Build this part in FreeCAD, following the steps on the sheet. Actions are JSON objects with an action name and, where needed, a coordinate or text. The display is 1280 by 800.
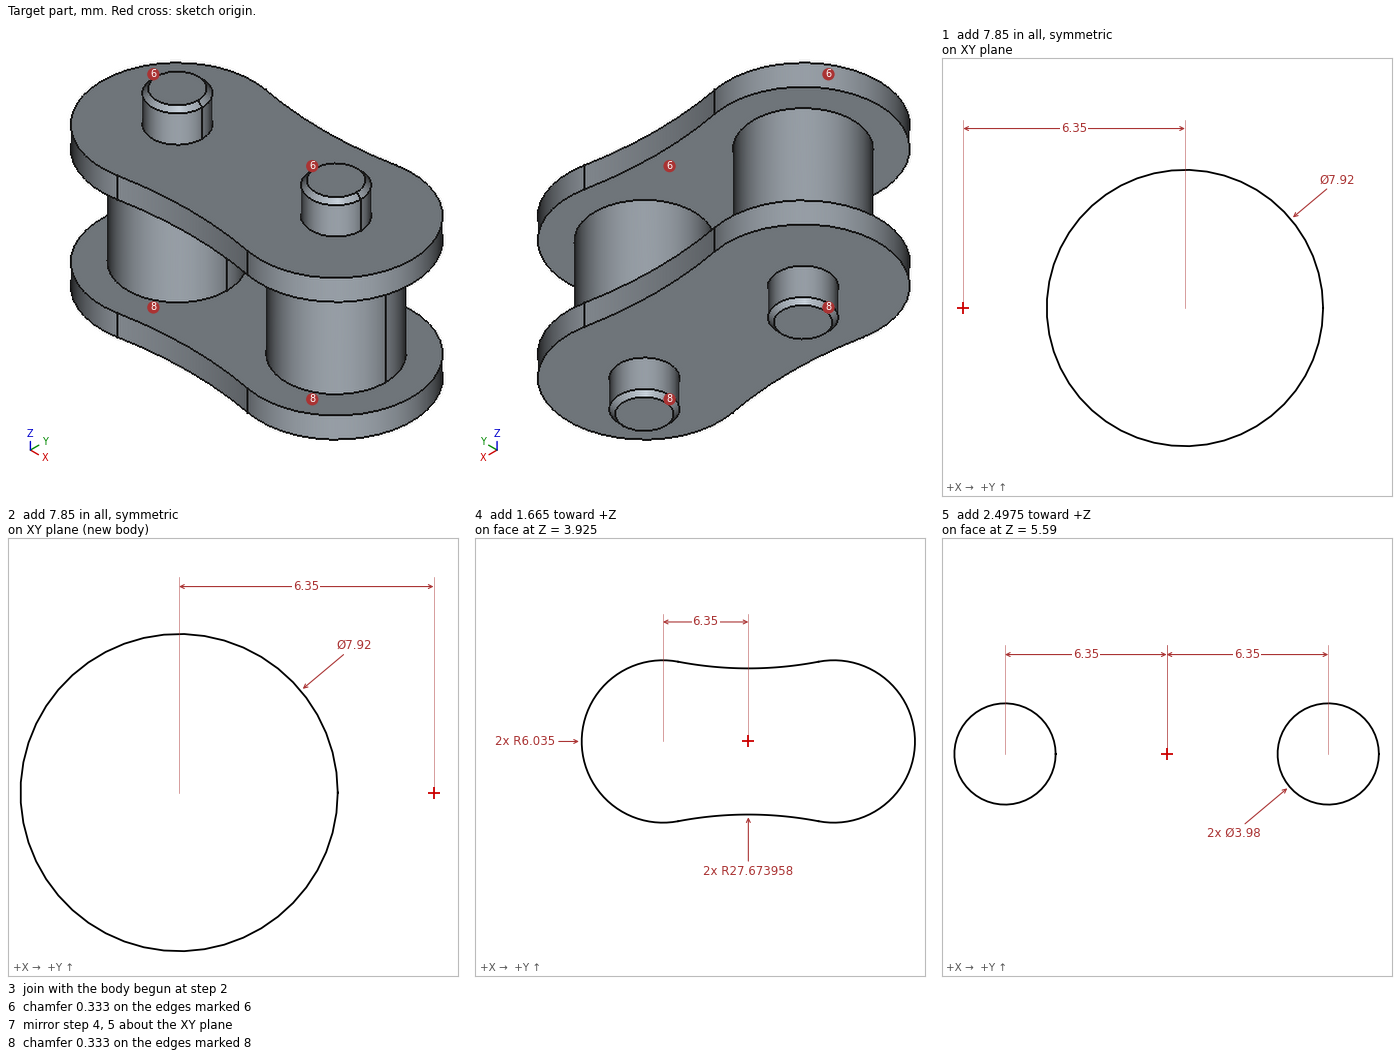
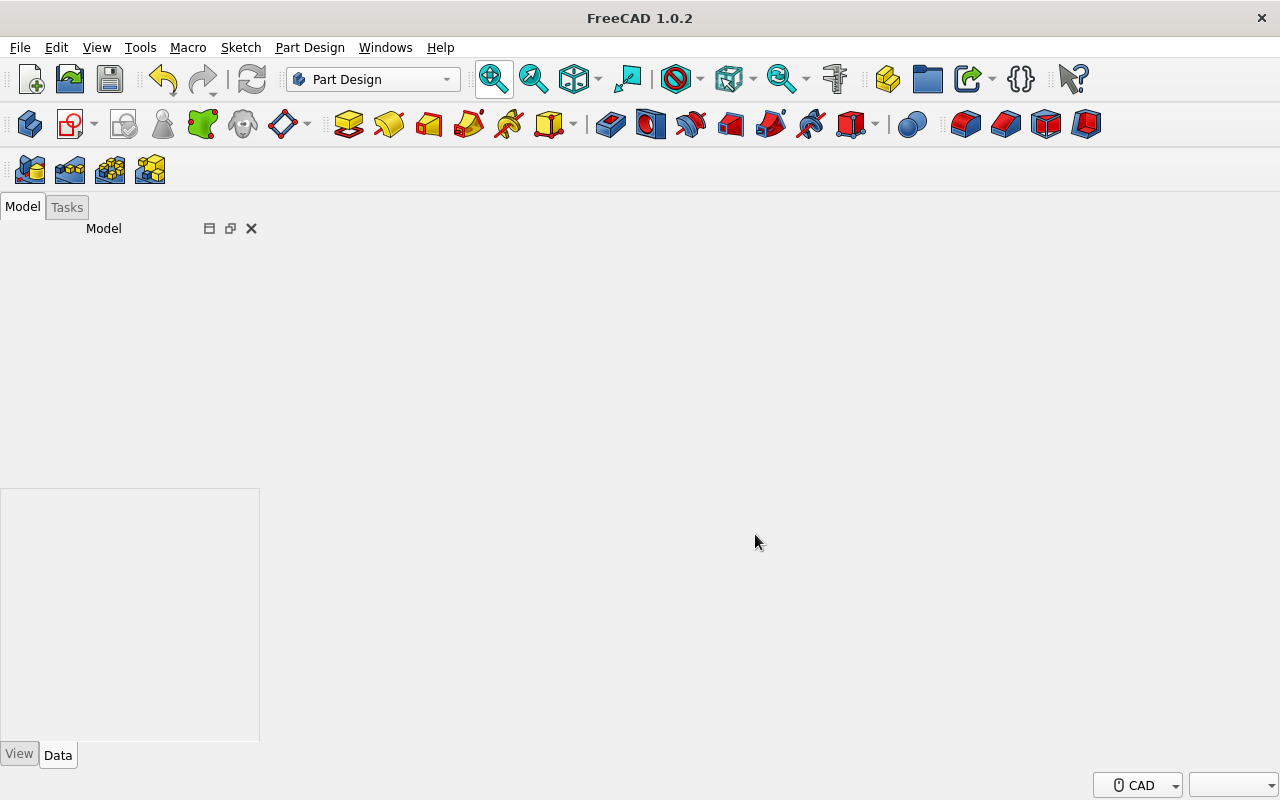
{"action": "left_click", "coordinate": [30, 80]}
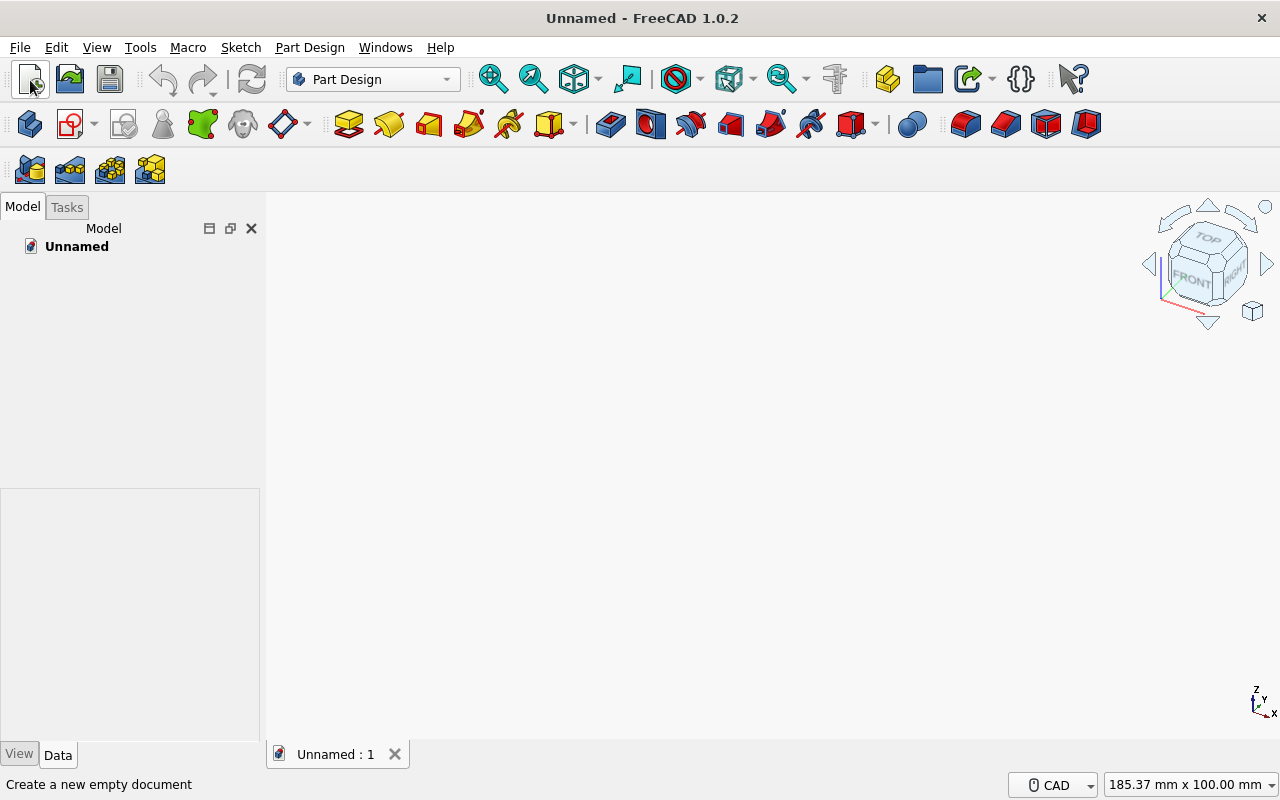
{"action": "left_click", "coordinate": [70, 124]}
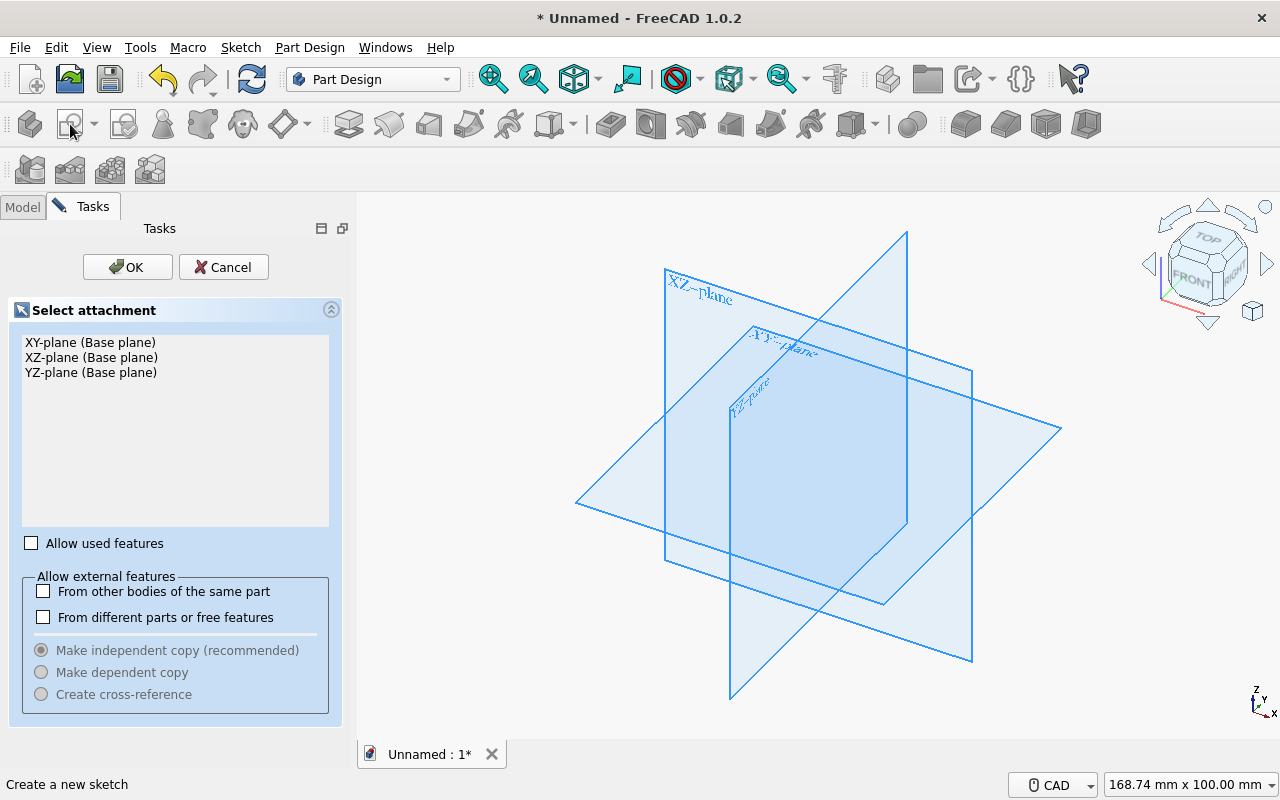
{"action": "left_click", "coordinate": [82, 342]}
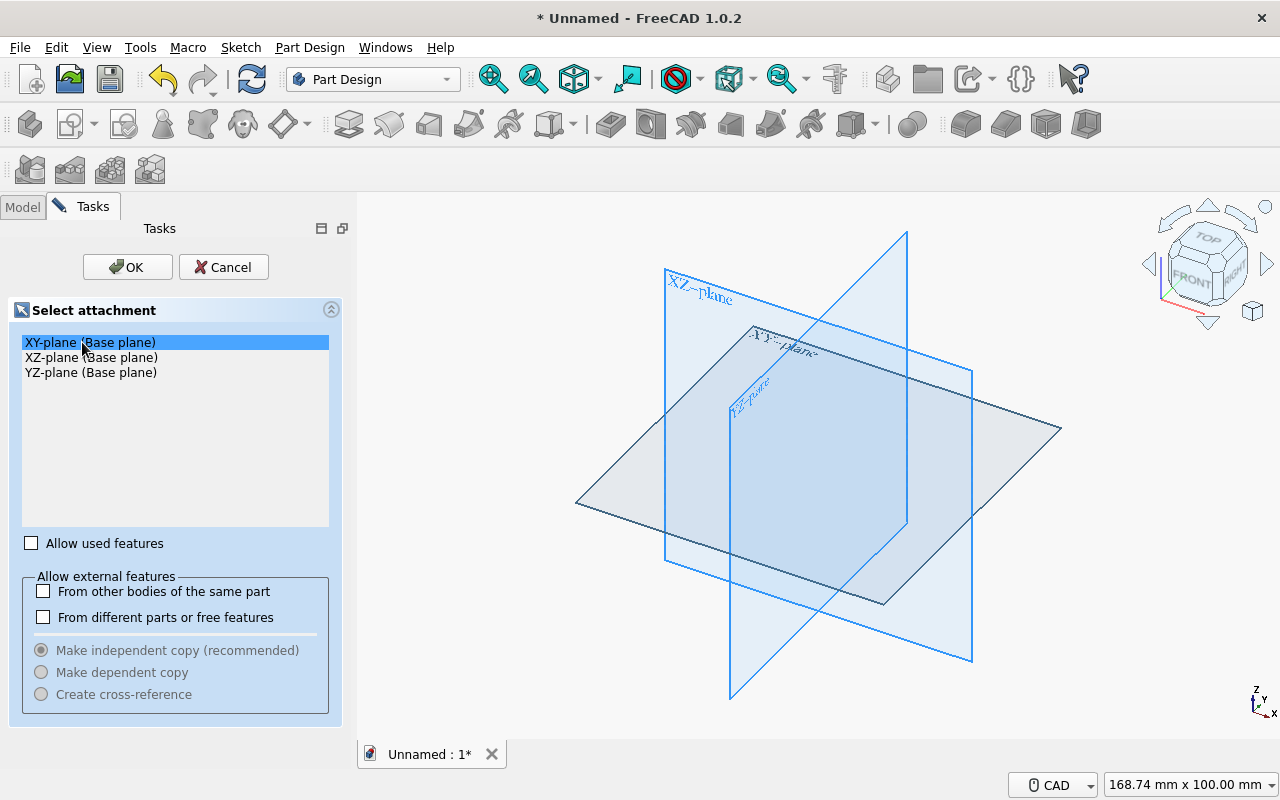
{"action": "left_click", "coordinate": [128, 267]}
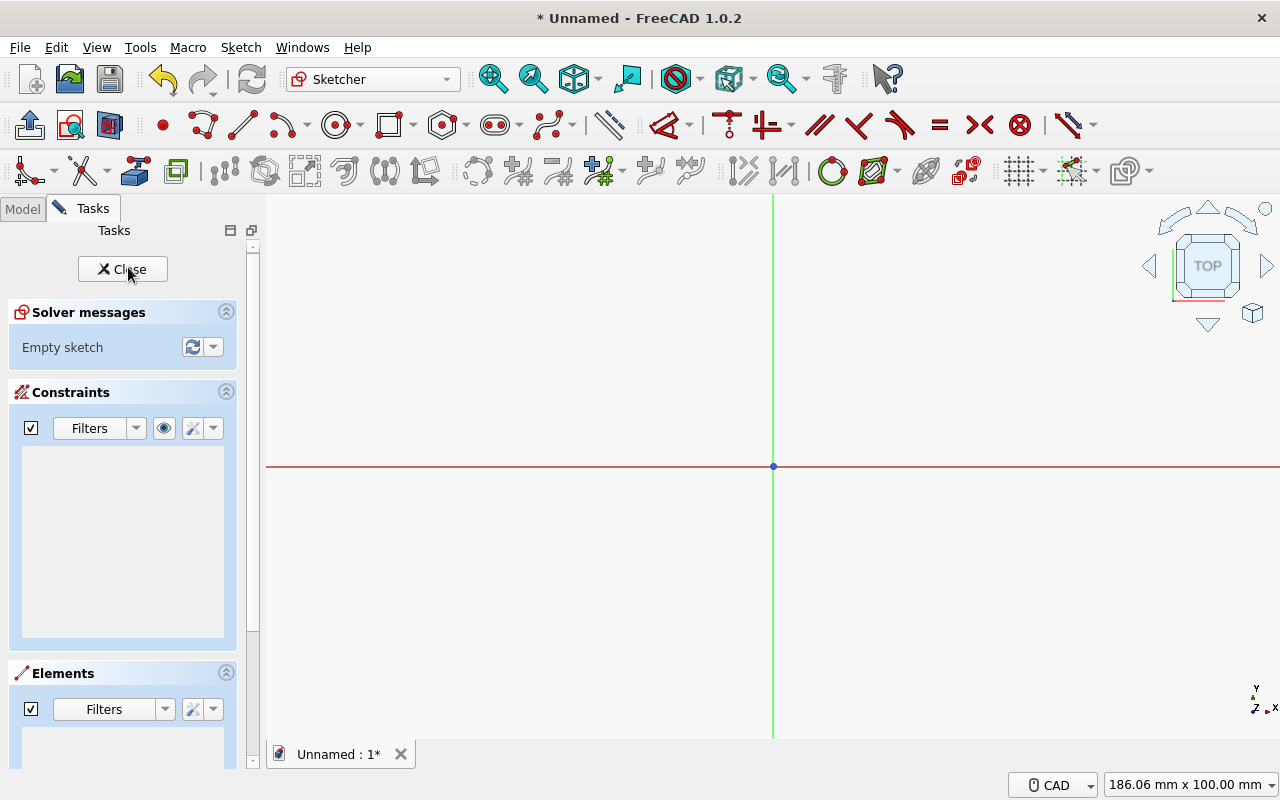
{"action": "scroll", "coordinate": [816, 466], "scroll_direction": "up", "scroll_amount": 10}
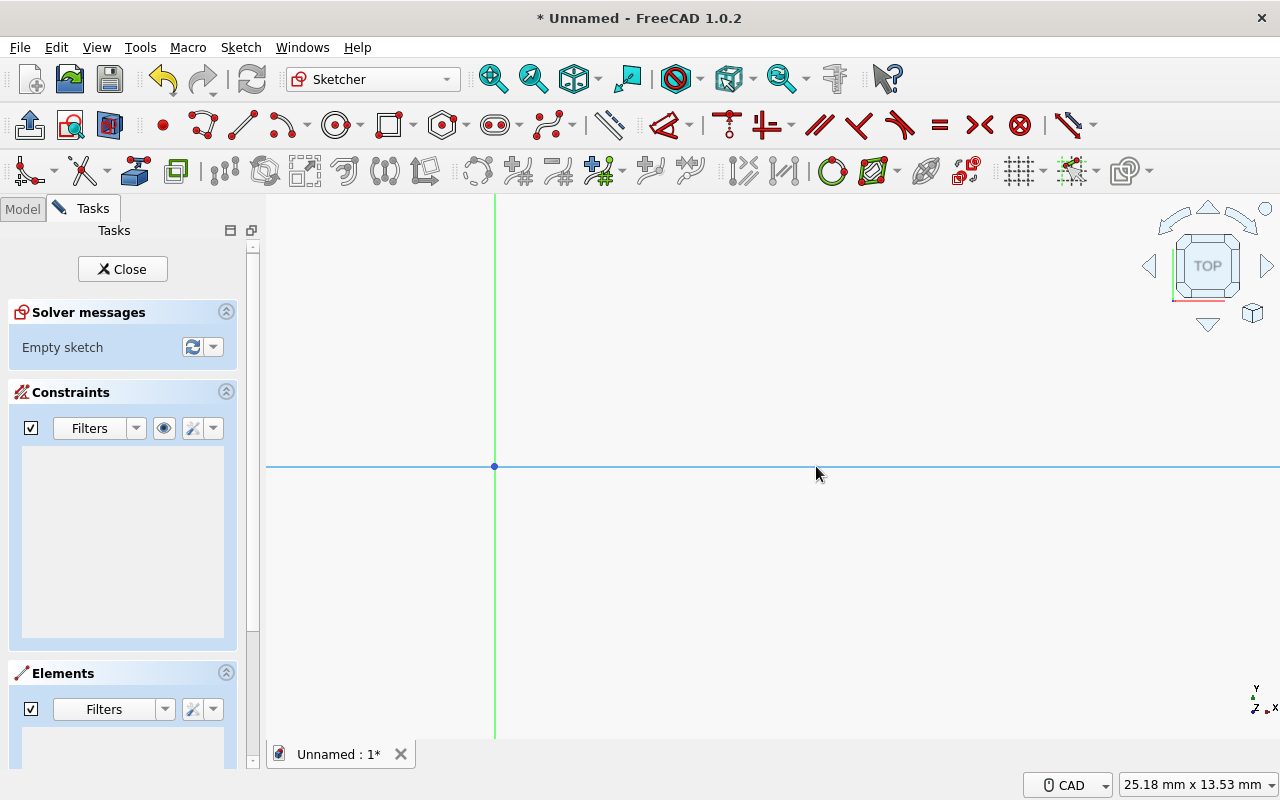
{"action": "left_click", "coordinate": [336, 126]}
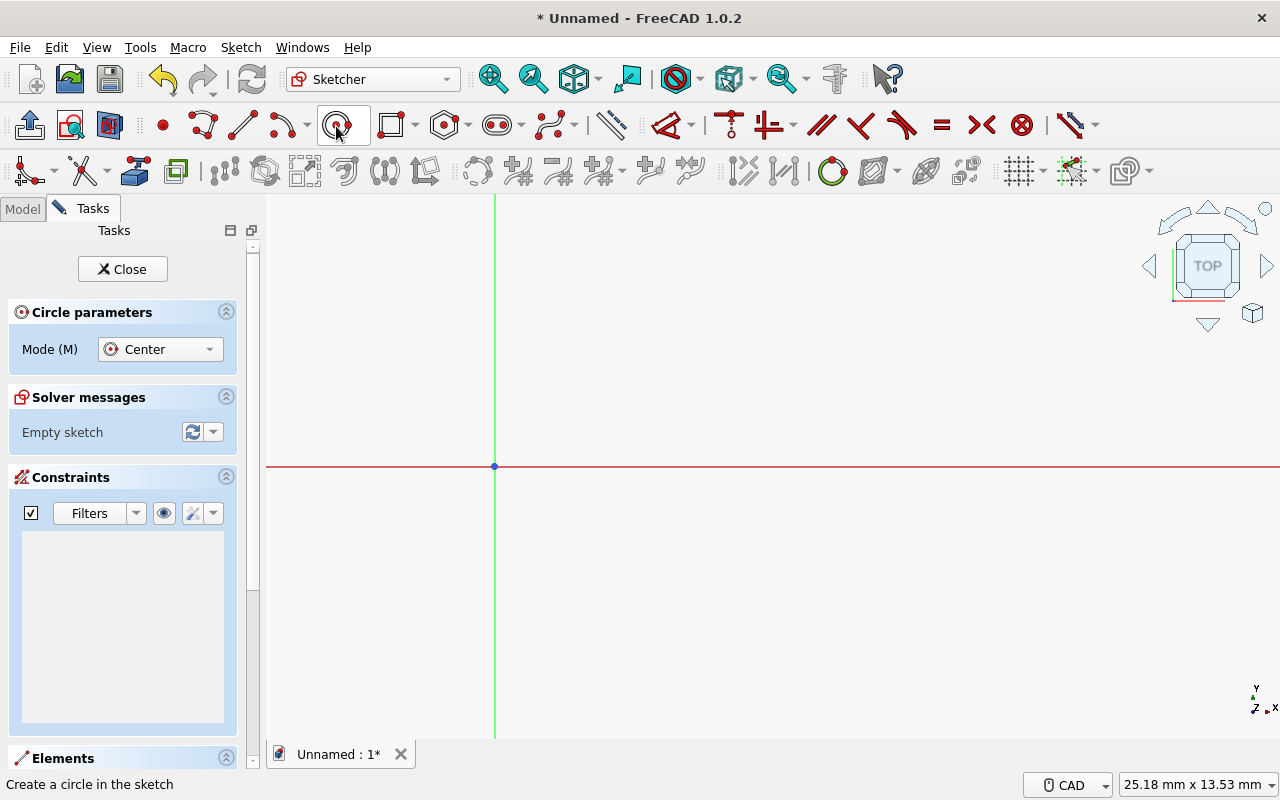
{"action": "left_click", "coordinate": [751, 466]}
{"action": "mouse_move", "coordinate": [863, 354]}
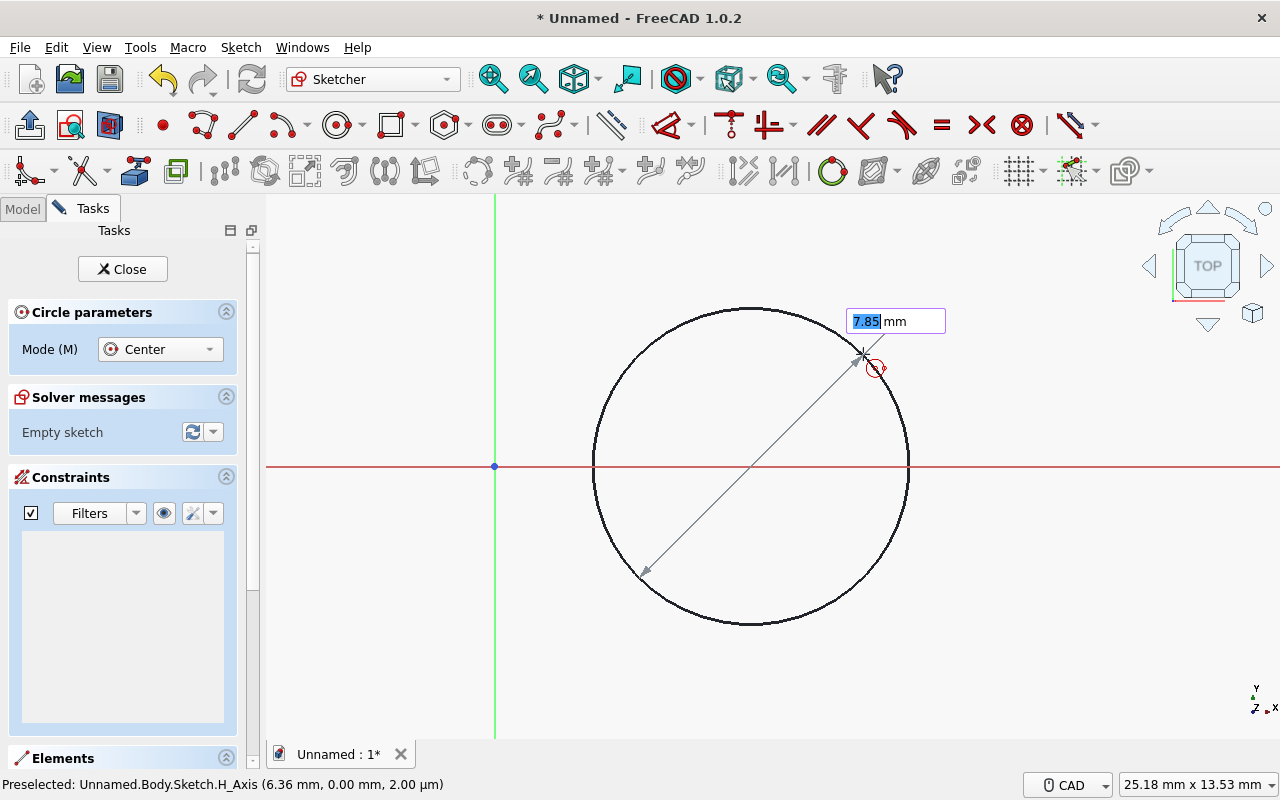
{"action": "type", "text": "7.92"}
{"action": "key", "text": "Return"}
{"action": "key", "text": "Escape"}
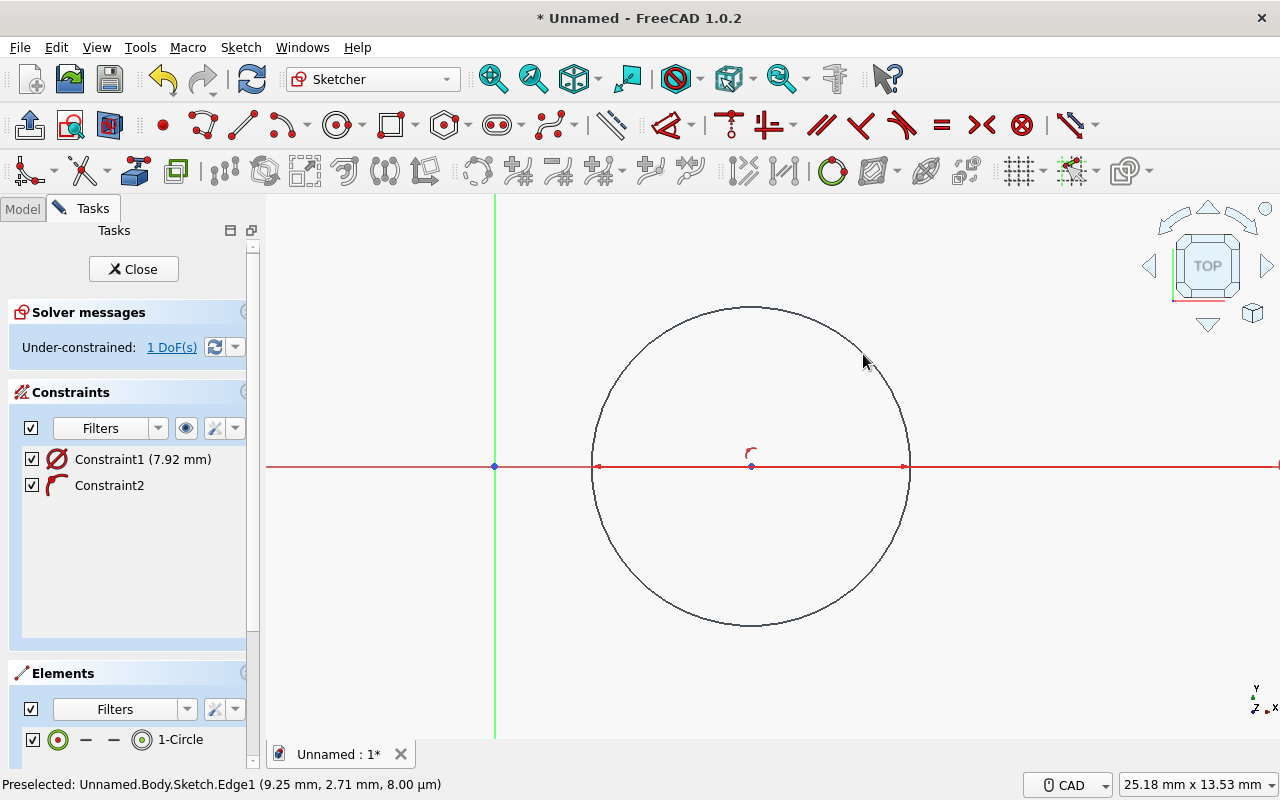
{"action": "left_click", "coordinate": [751, 466]}